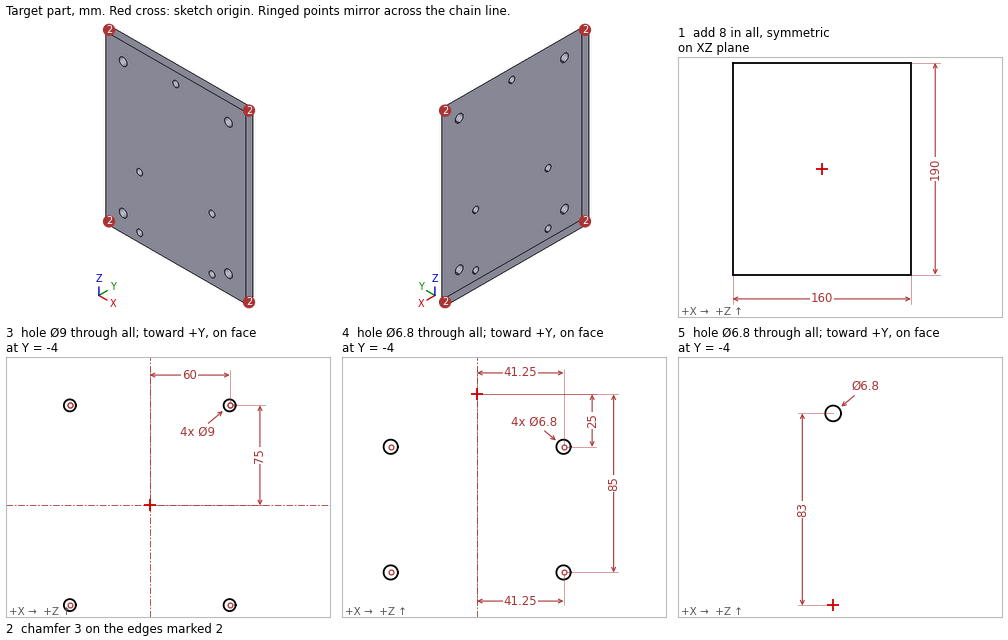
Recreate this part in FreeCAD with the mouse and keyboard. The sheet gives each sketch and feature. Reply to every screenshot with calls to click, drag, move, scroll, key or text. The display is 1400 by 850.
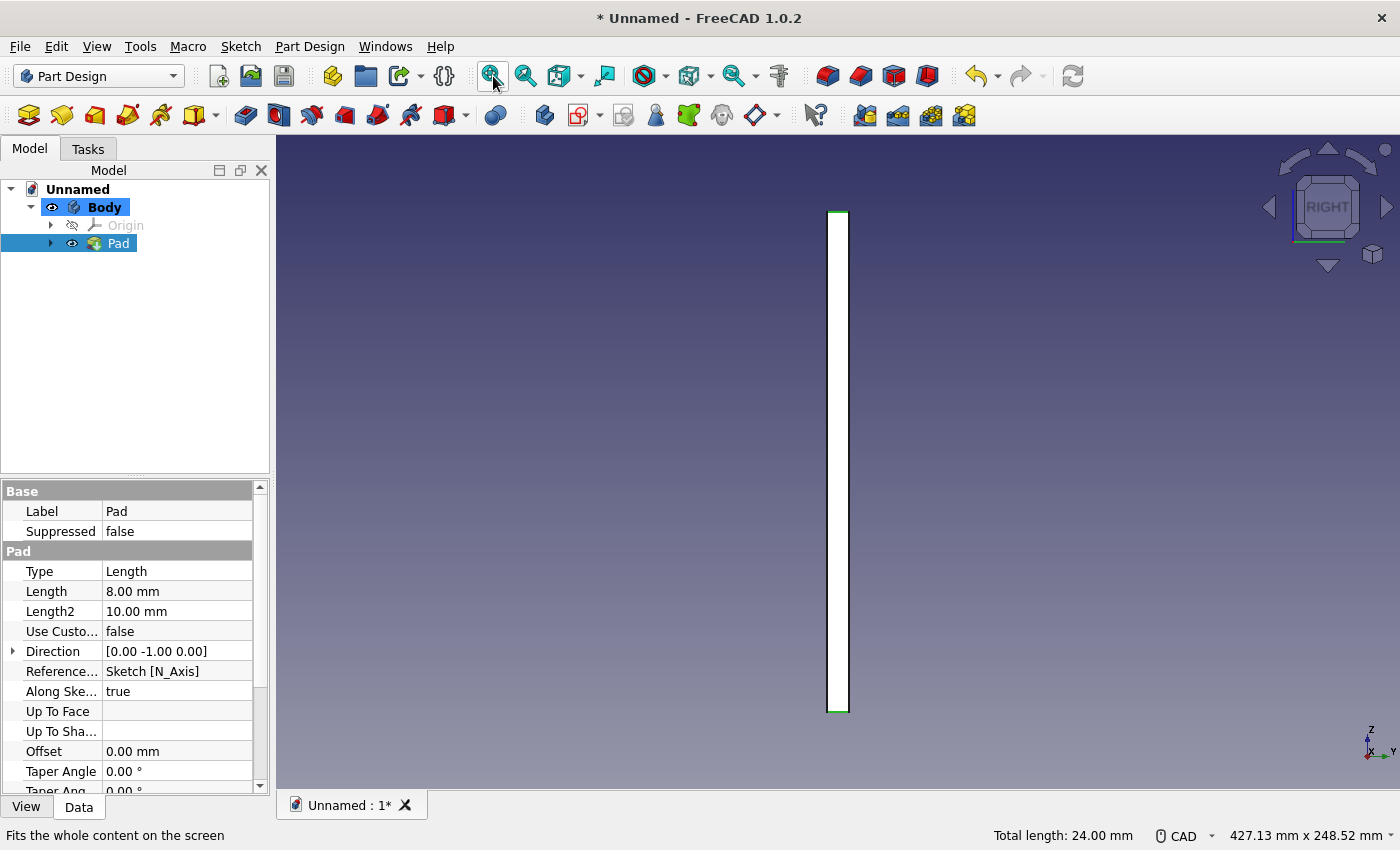
key(5)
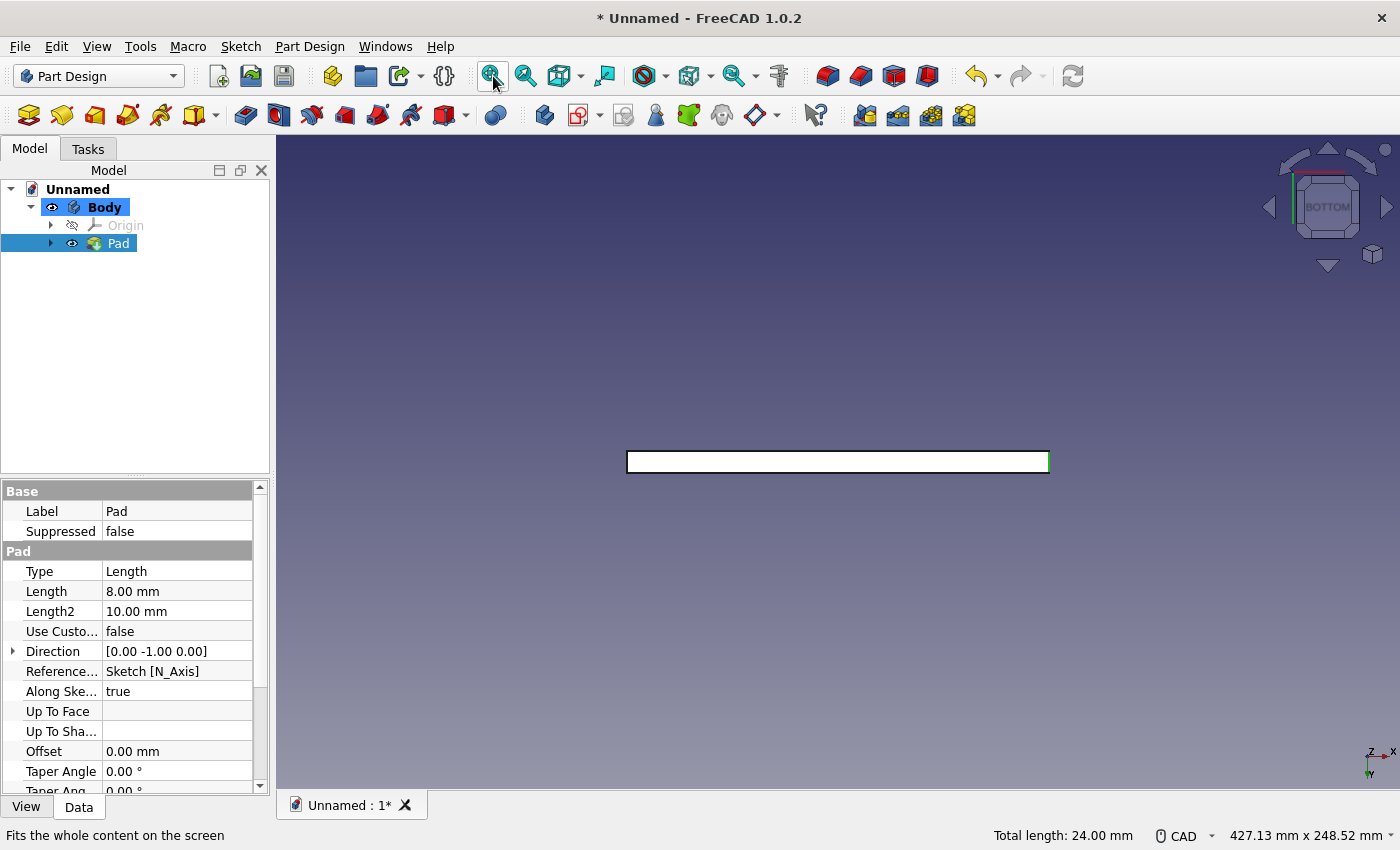
click(493, 76)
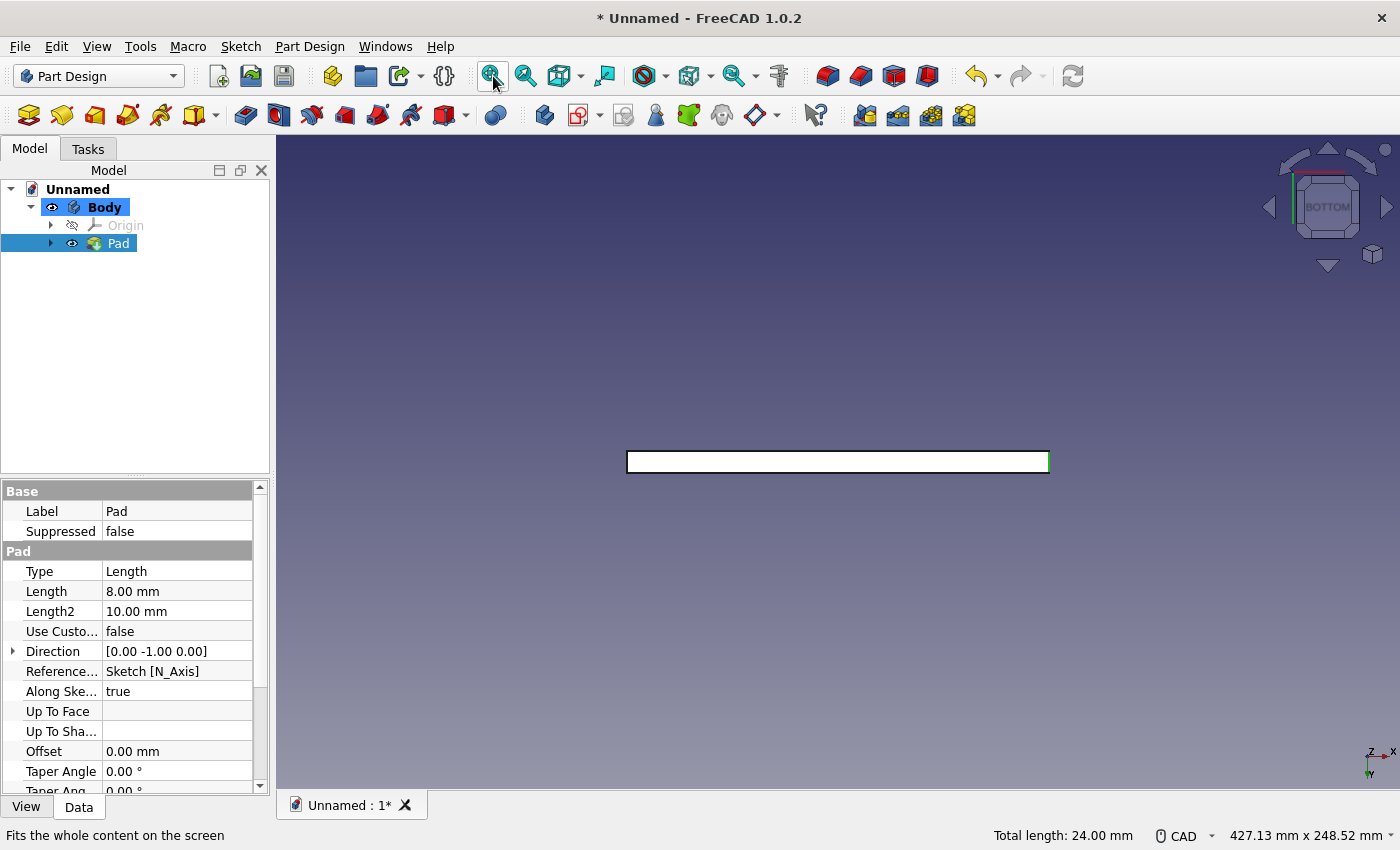
click(627, 461, ctrl)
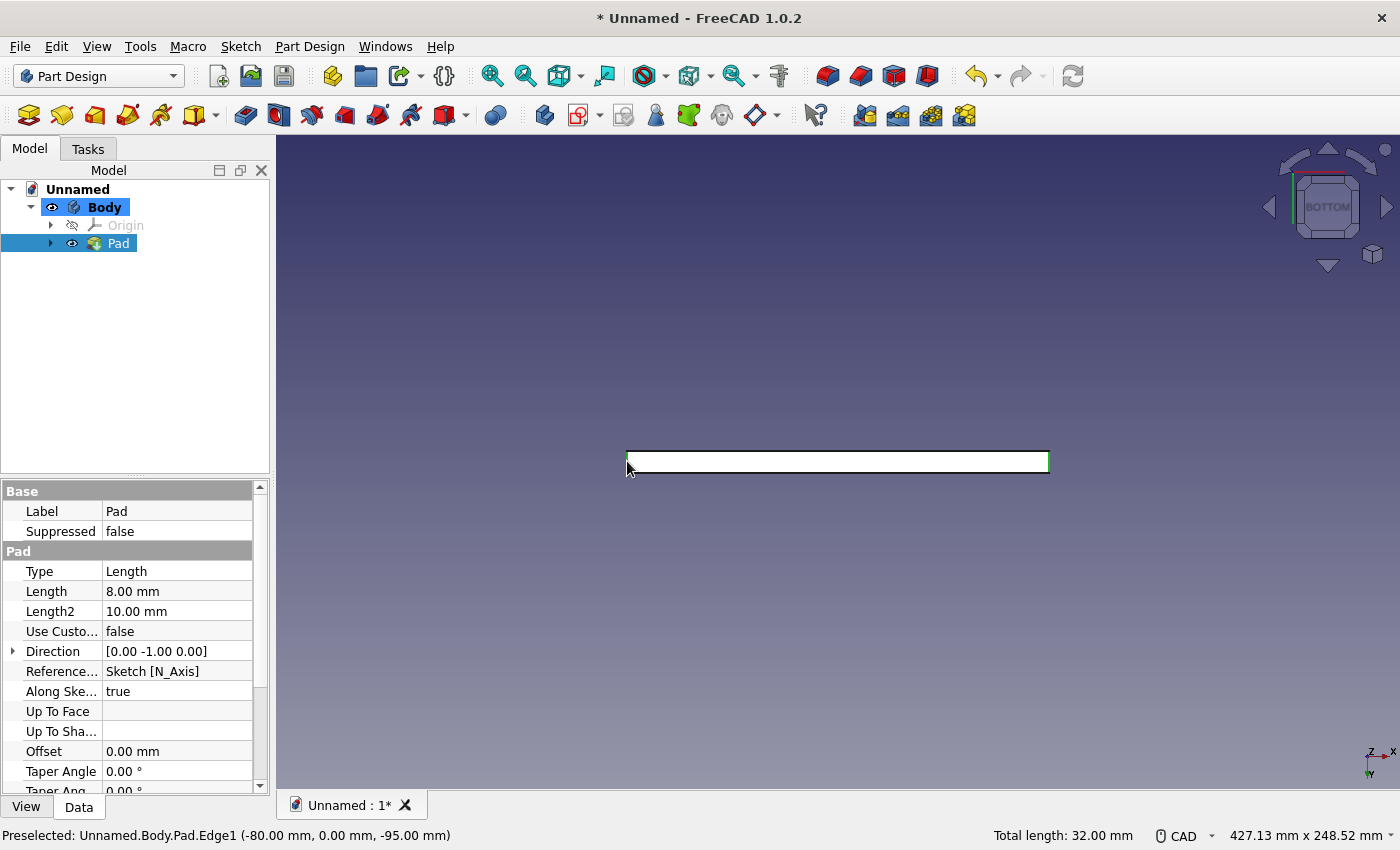
click(861, 76)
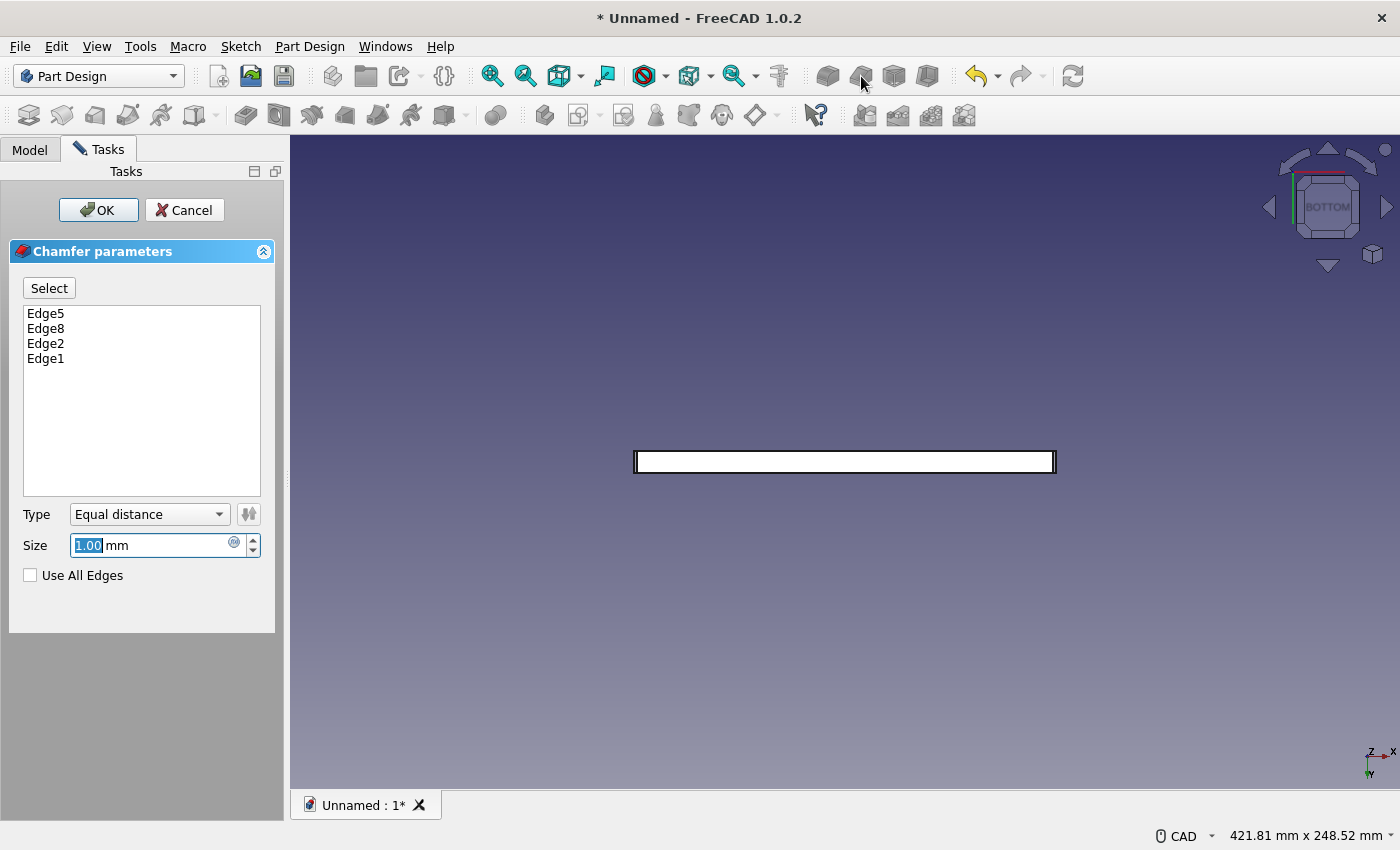
text(3)
key(Tab)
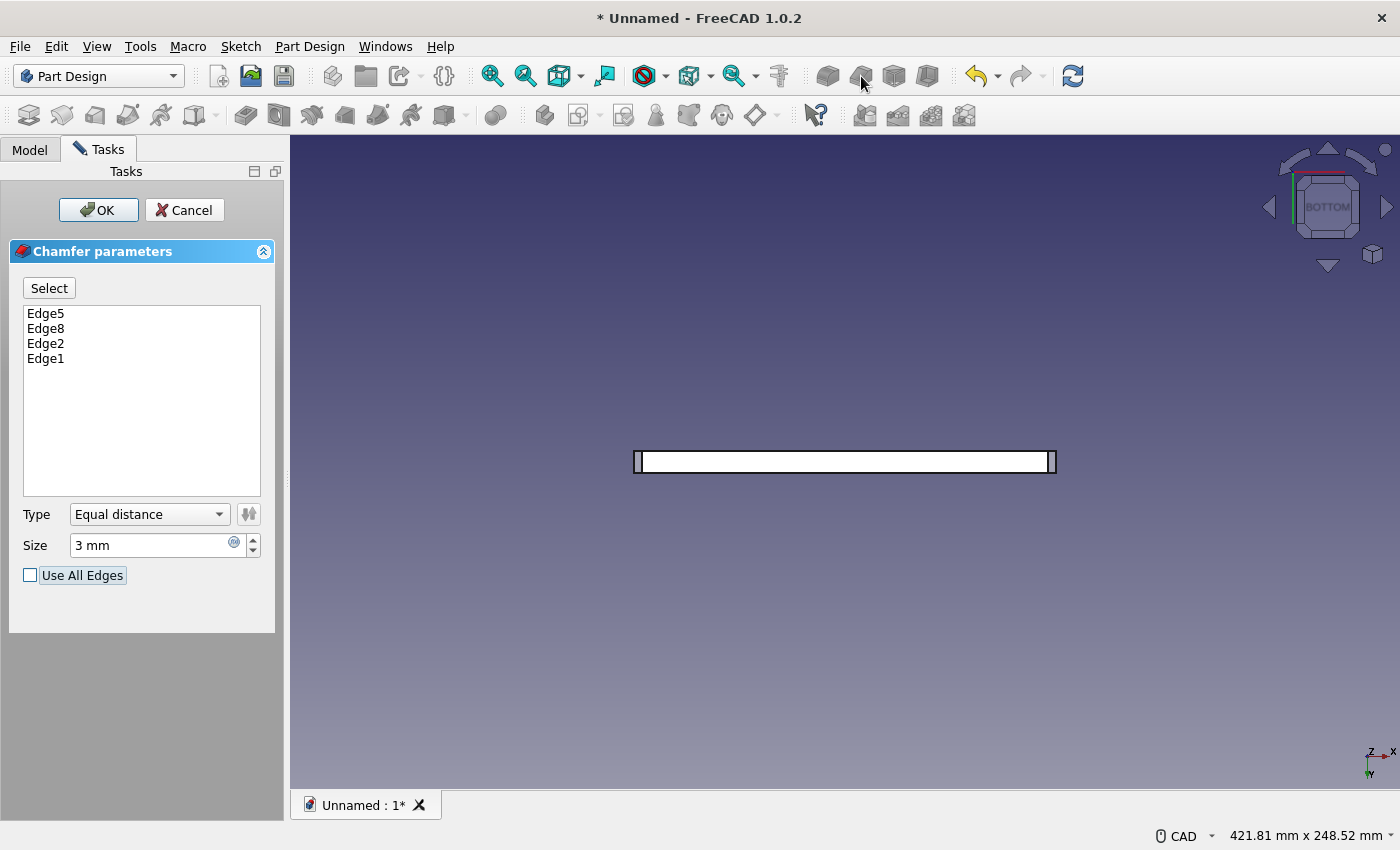
click(99, 210)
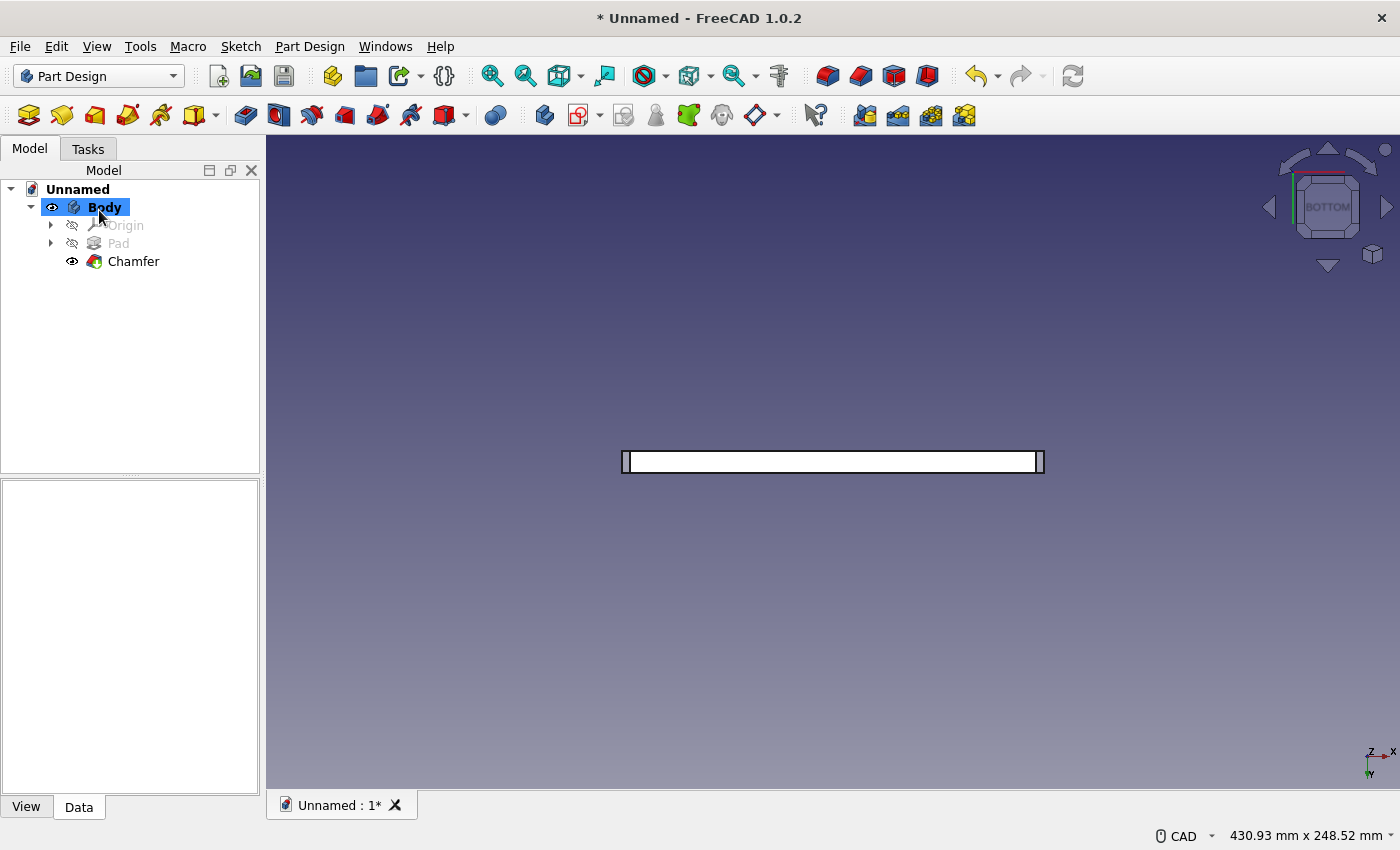
click(493, 76)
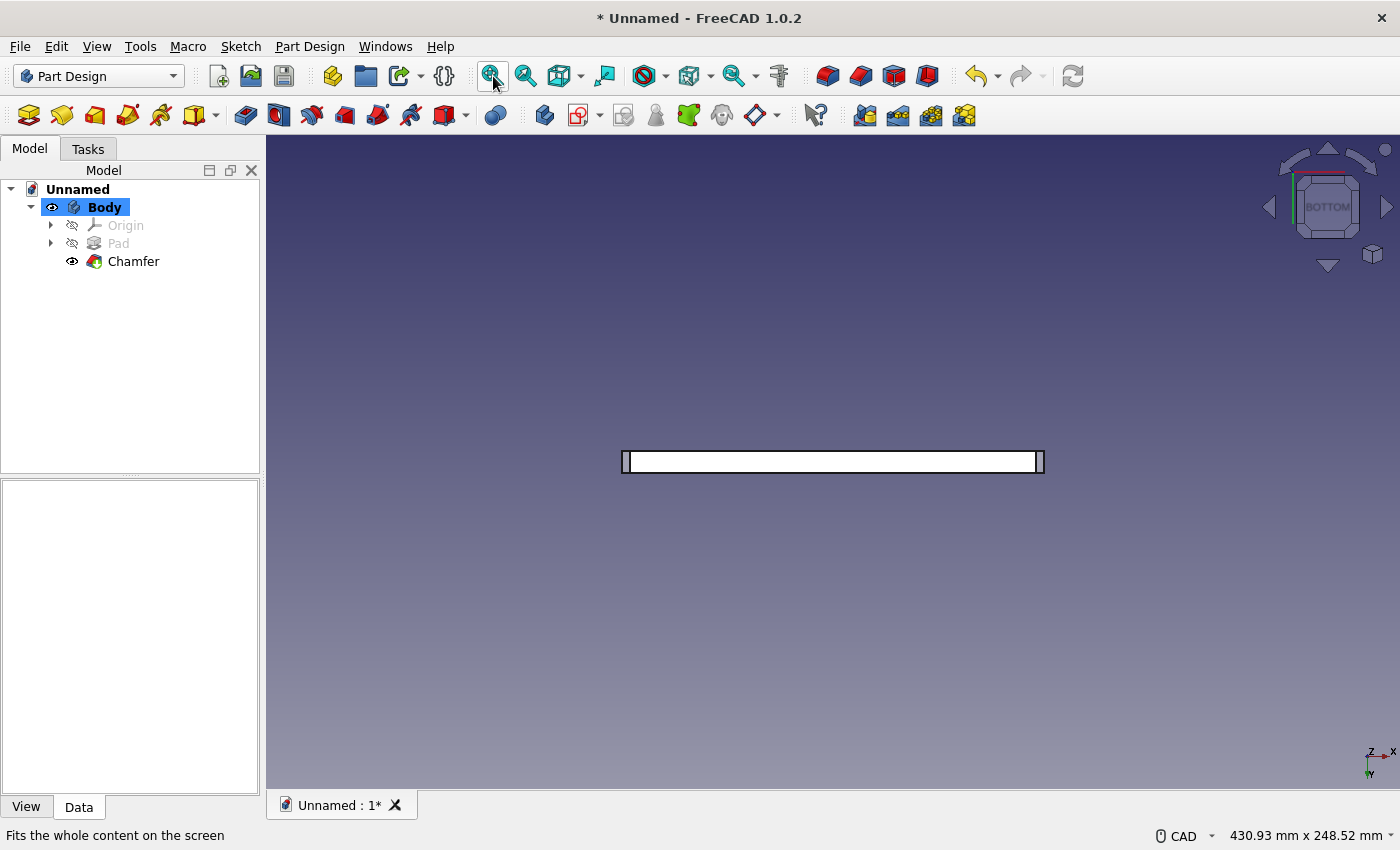
key(0)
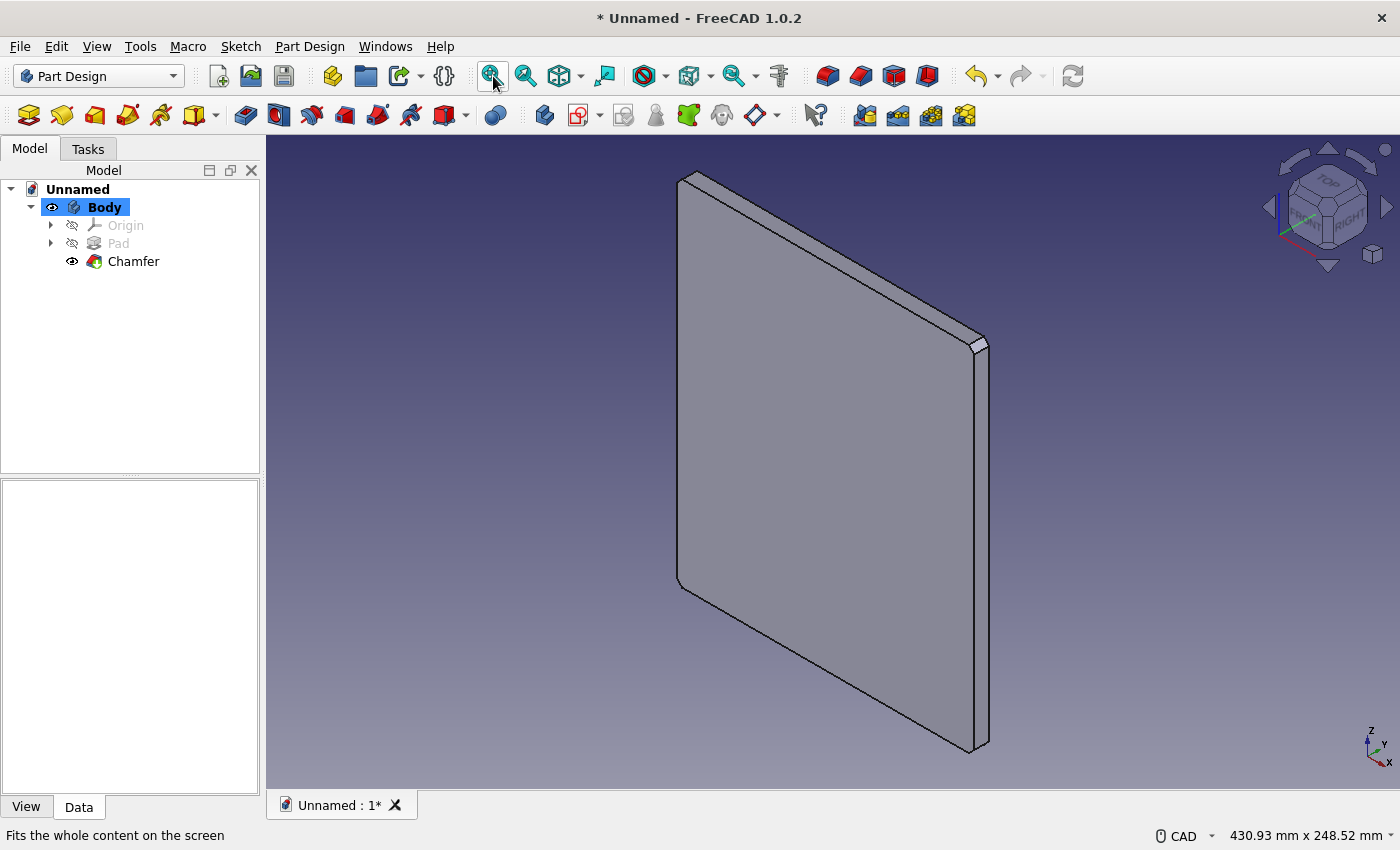
click(826, 465)